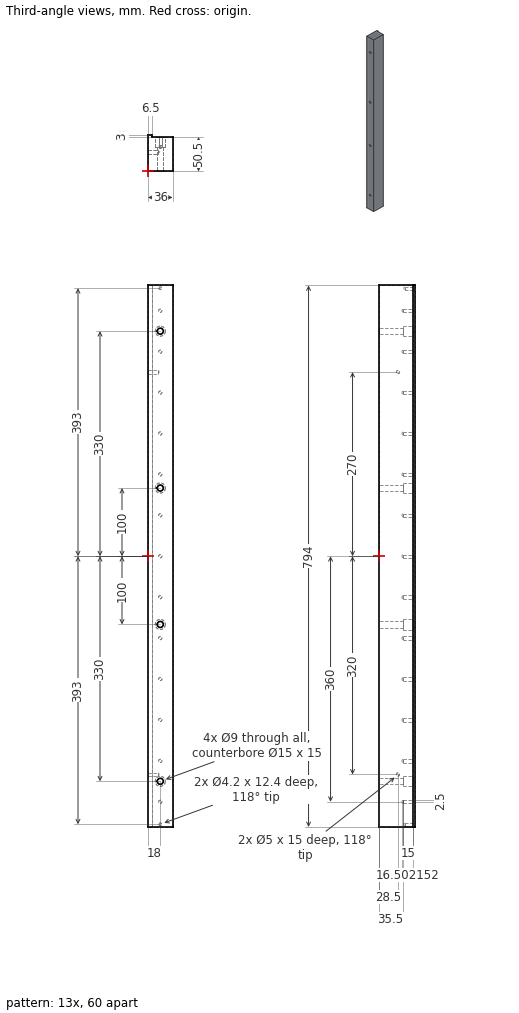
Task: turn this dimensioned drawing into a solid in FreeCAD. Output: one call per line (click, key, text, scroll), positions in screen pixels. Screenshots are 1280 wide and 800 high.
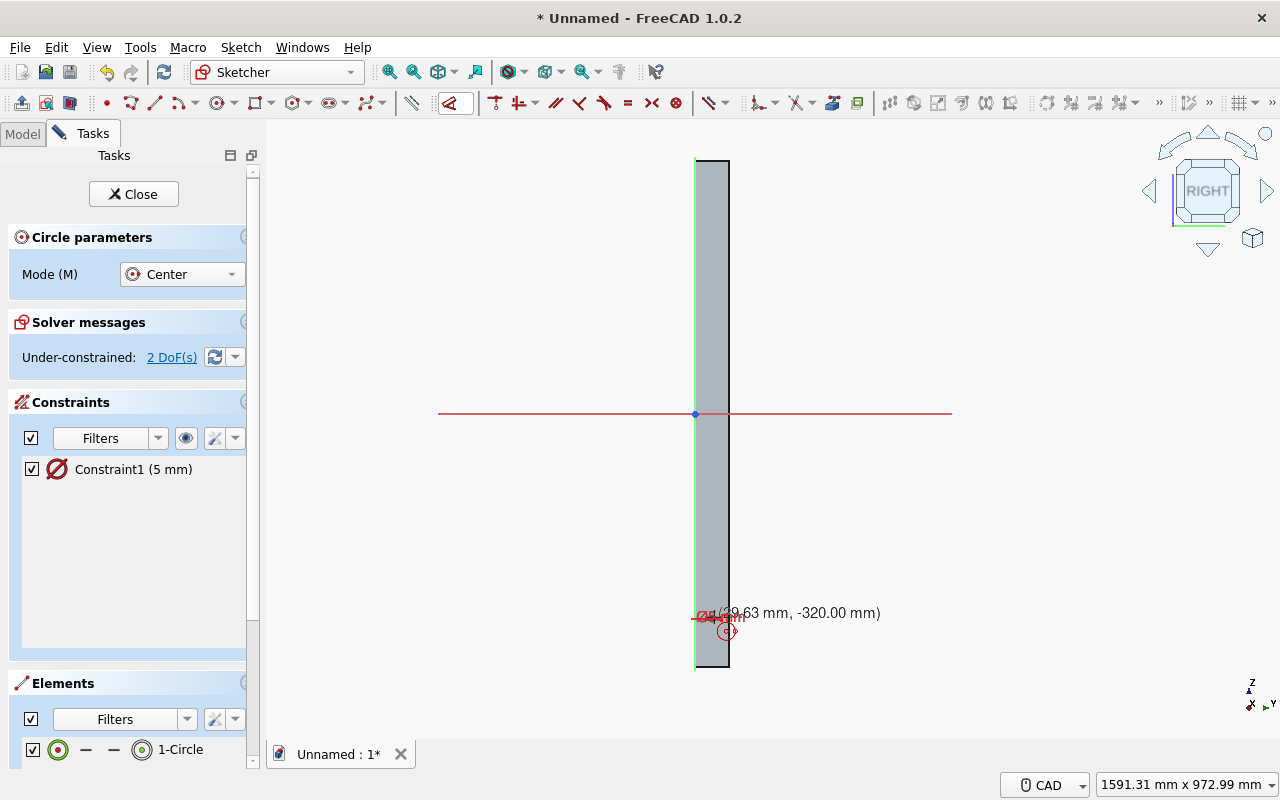
scroll(713, 242, up, 14)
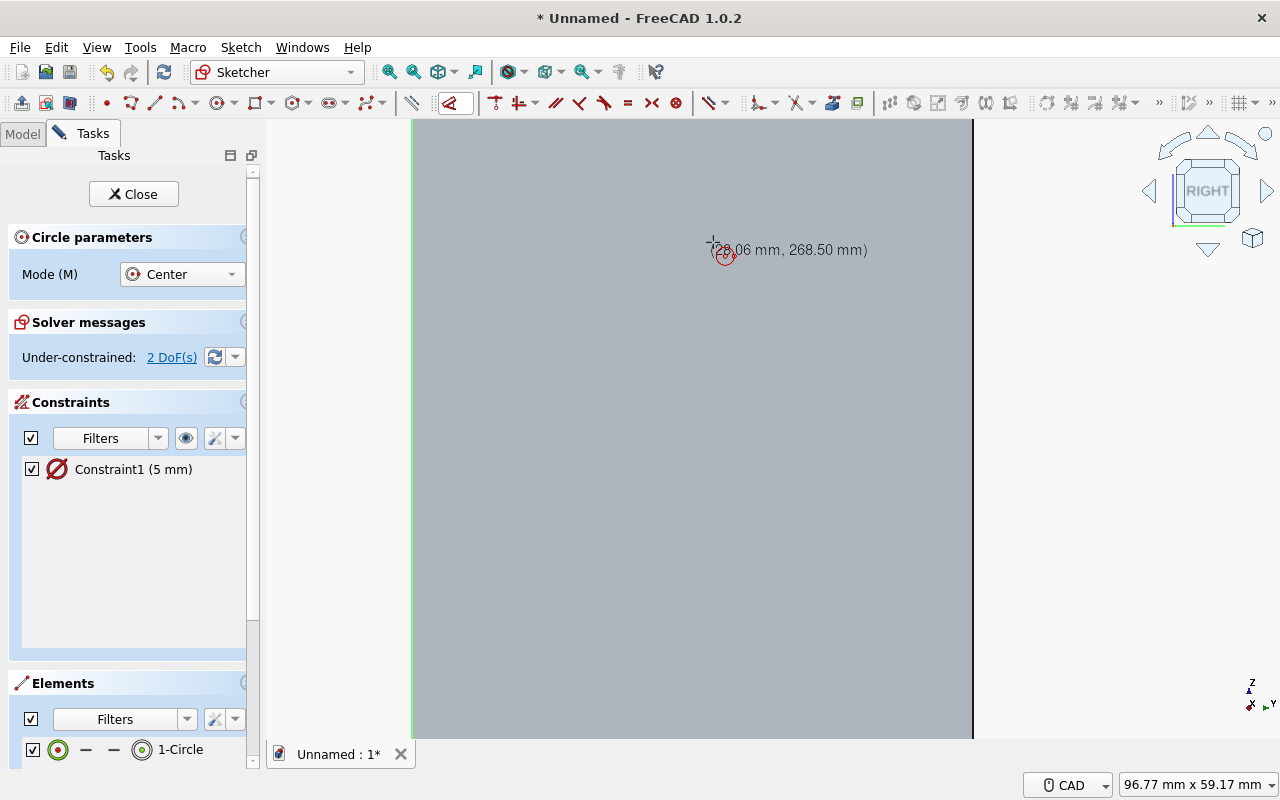
scroll(713, 241, down, 14)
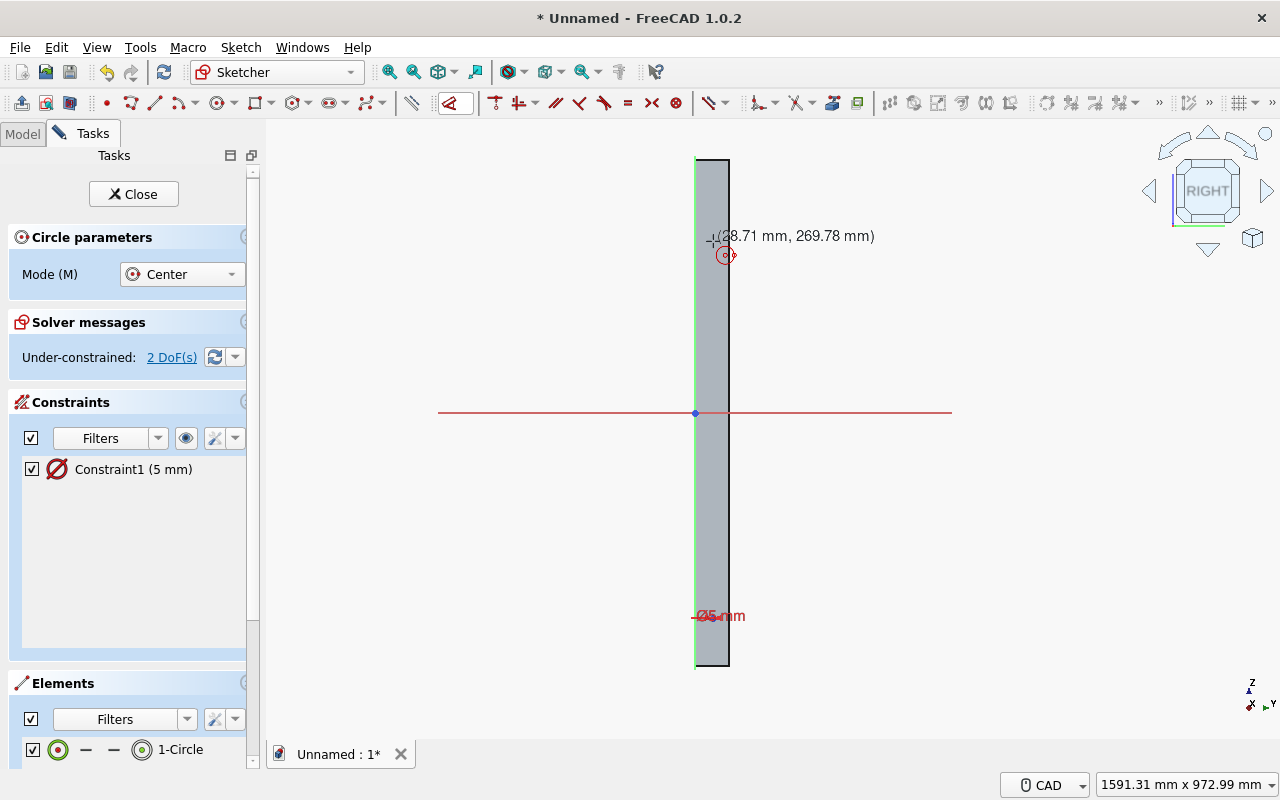
click(713, 241)
move(714, 240)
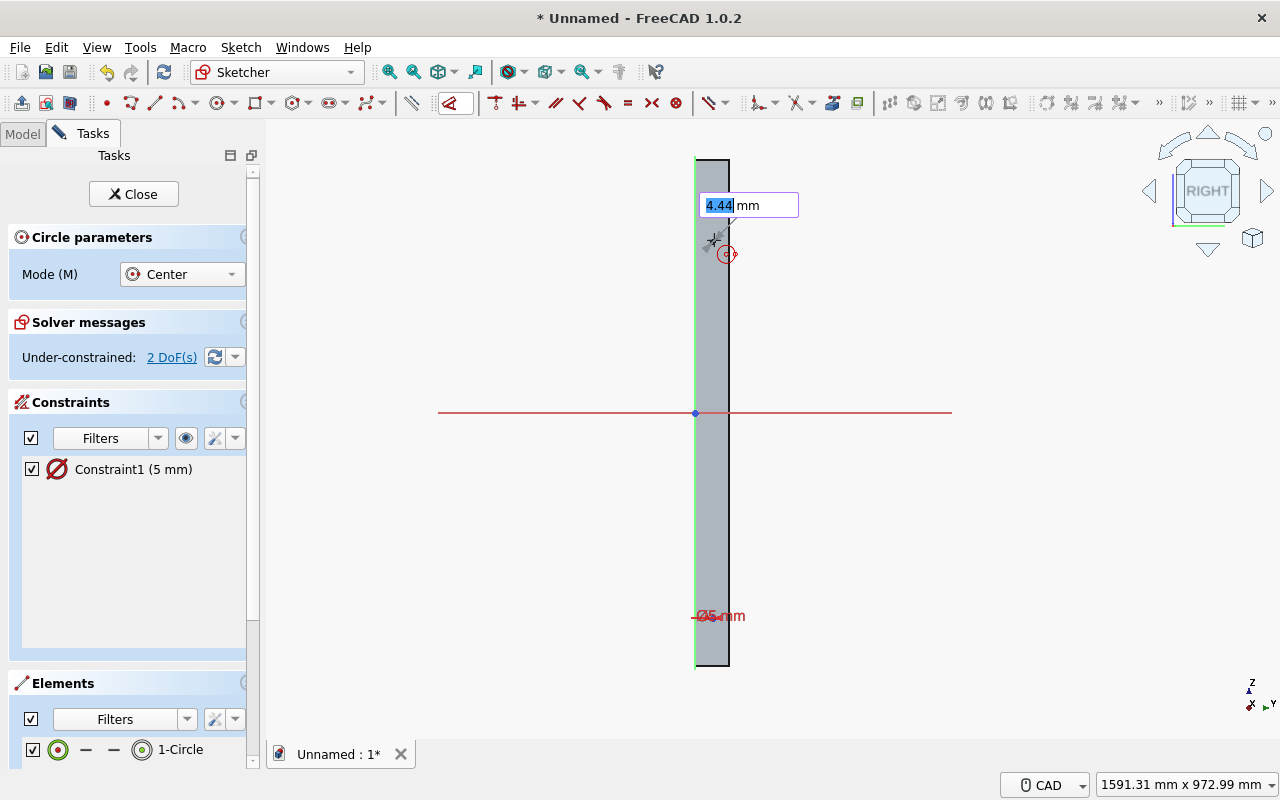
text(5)
key(Return)
key(Escape)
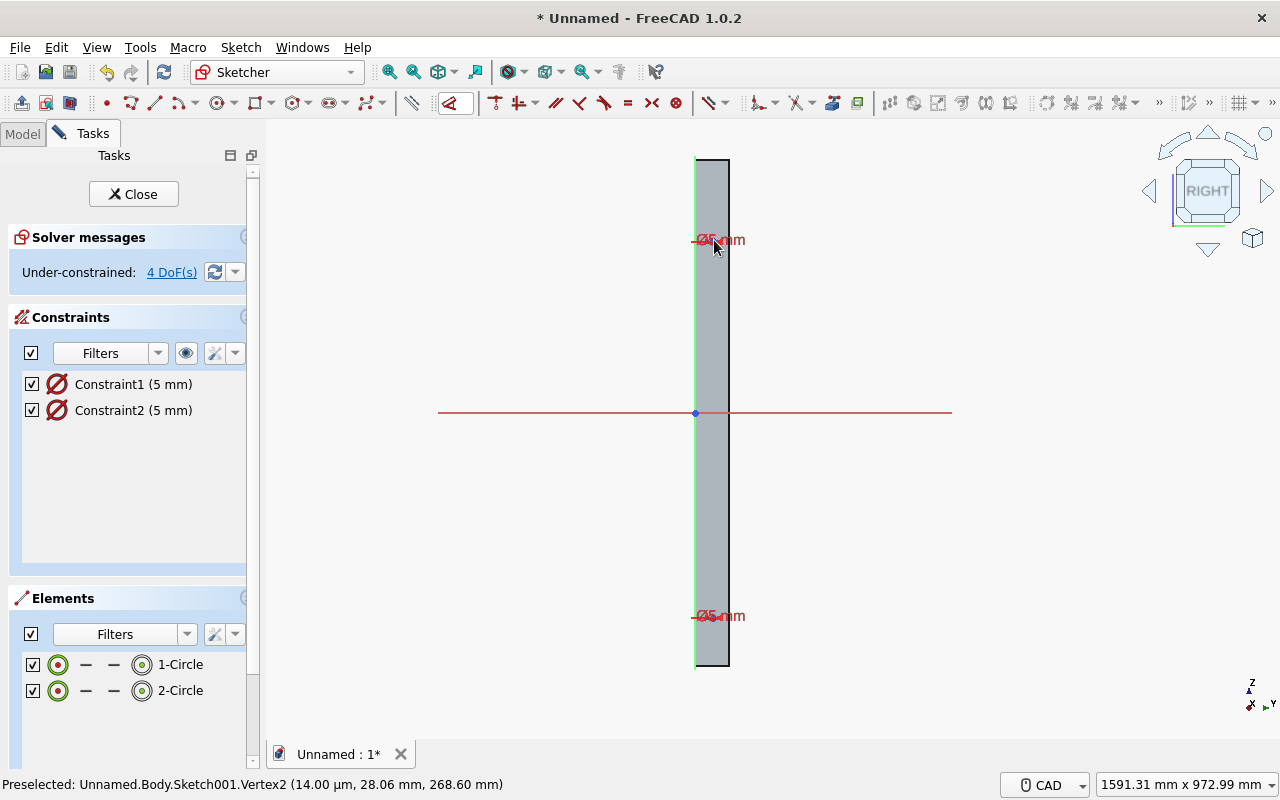
click(713, 618)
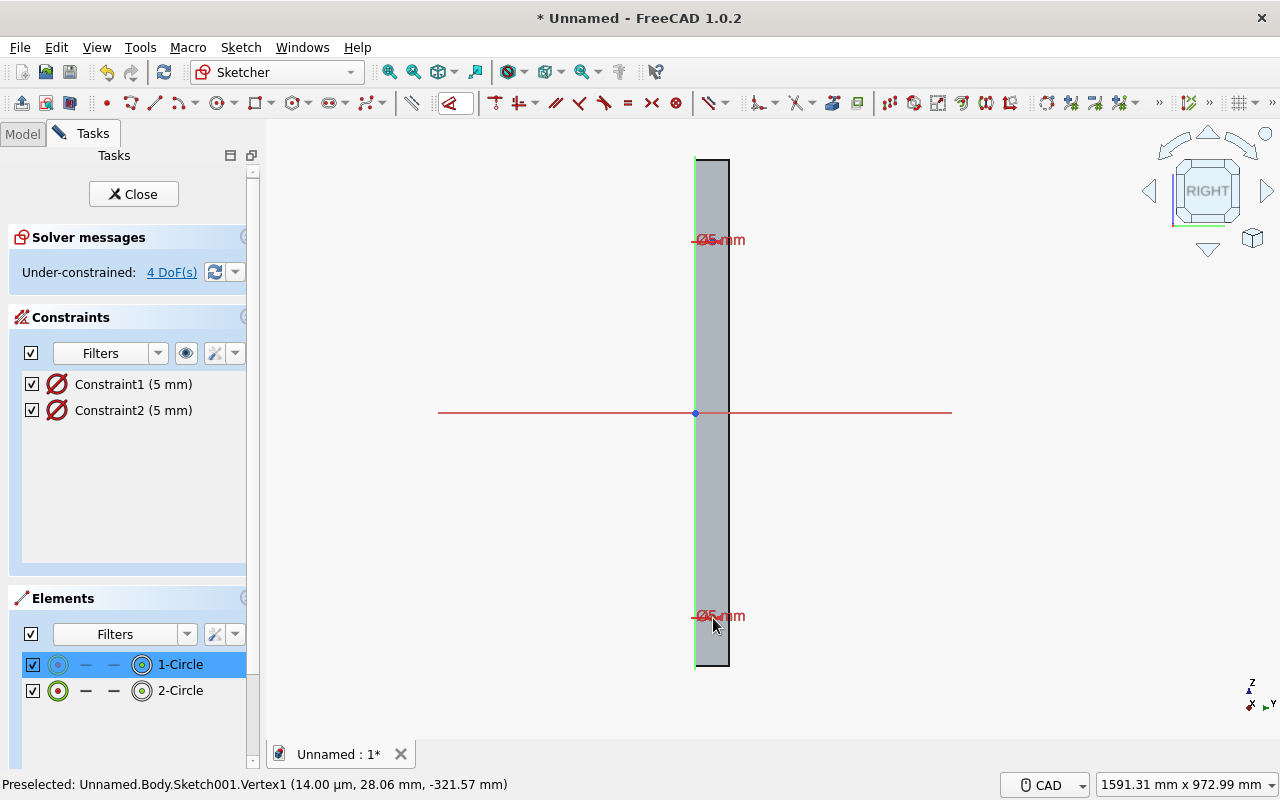
click(713, 242)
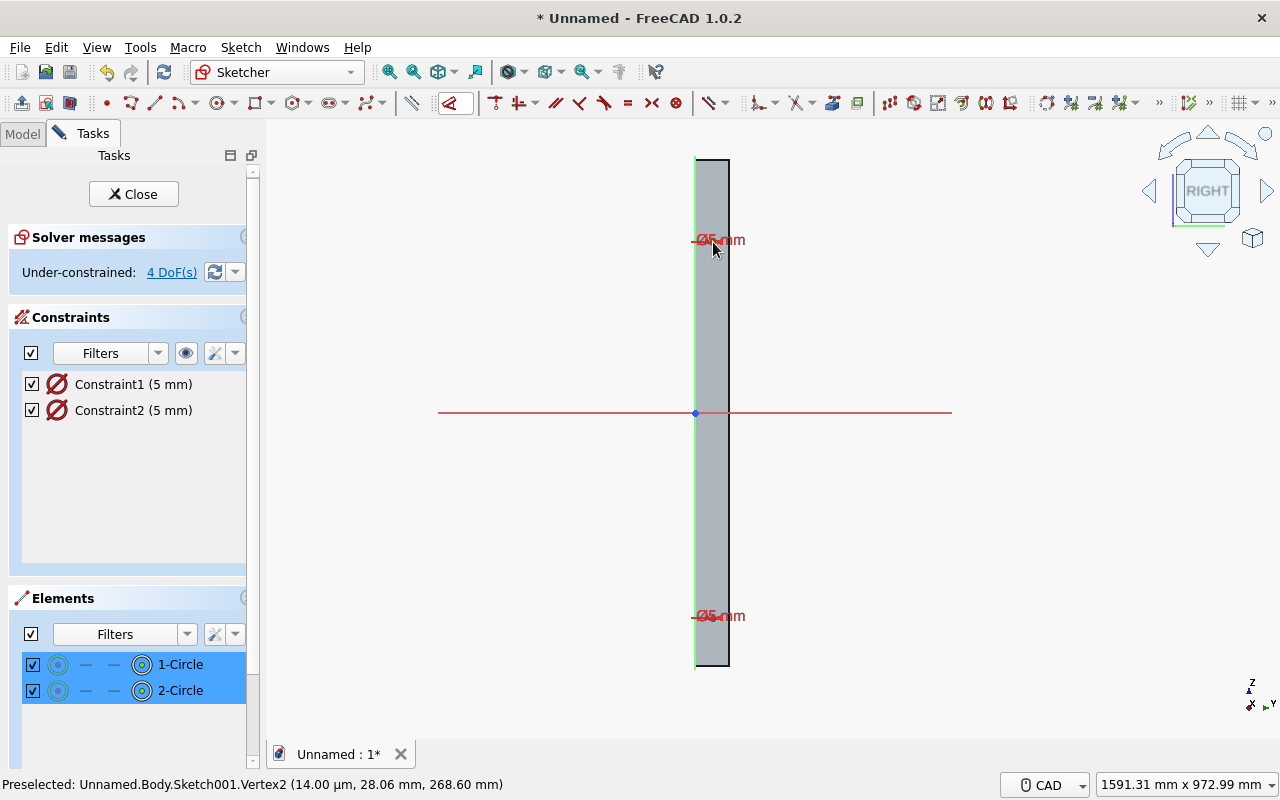
key(v)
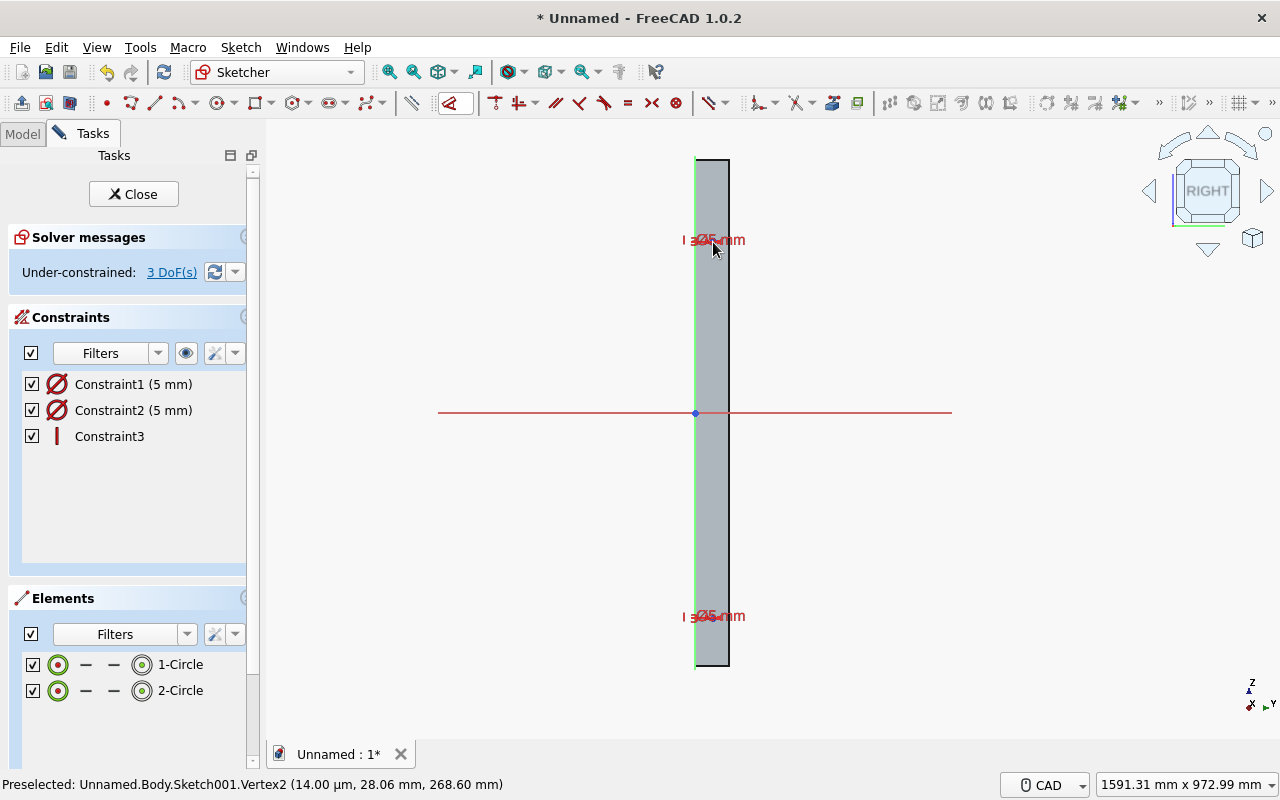
click(713, 618)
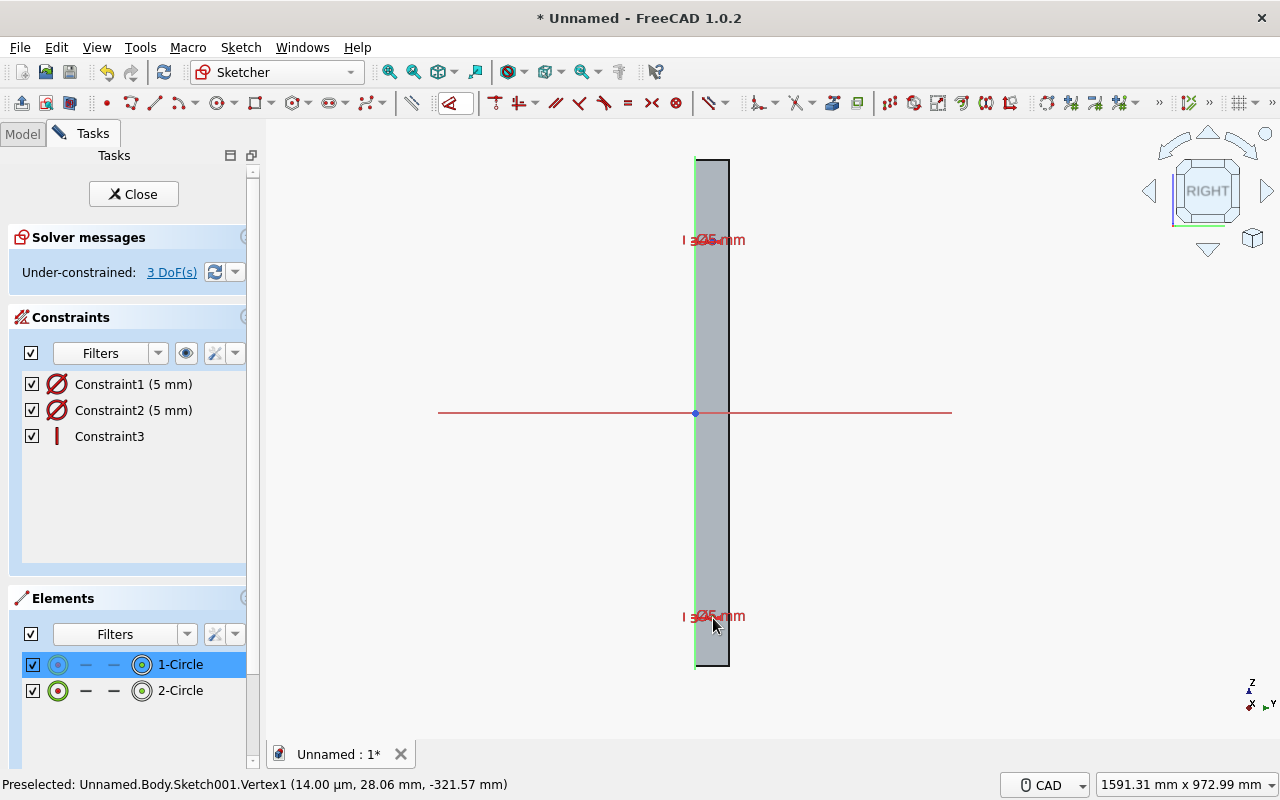
key(i)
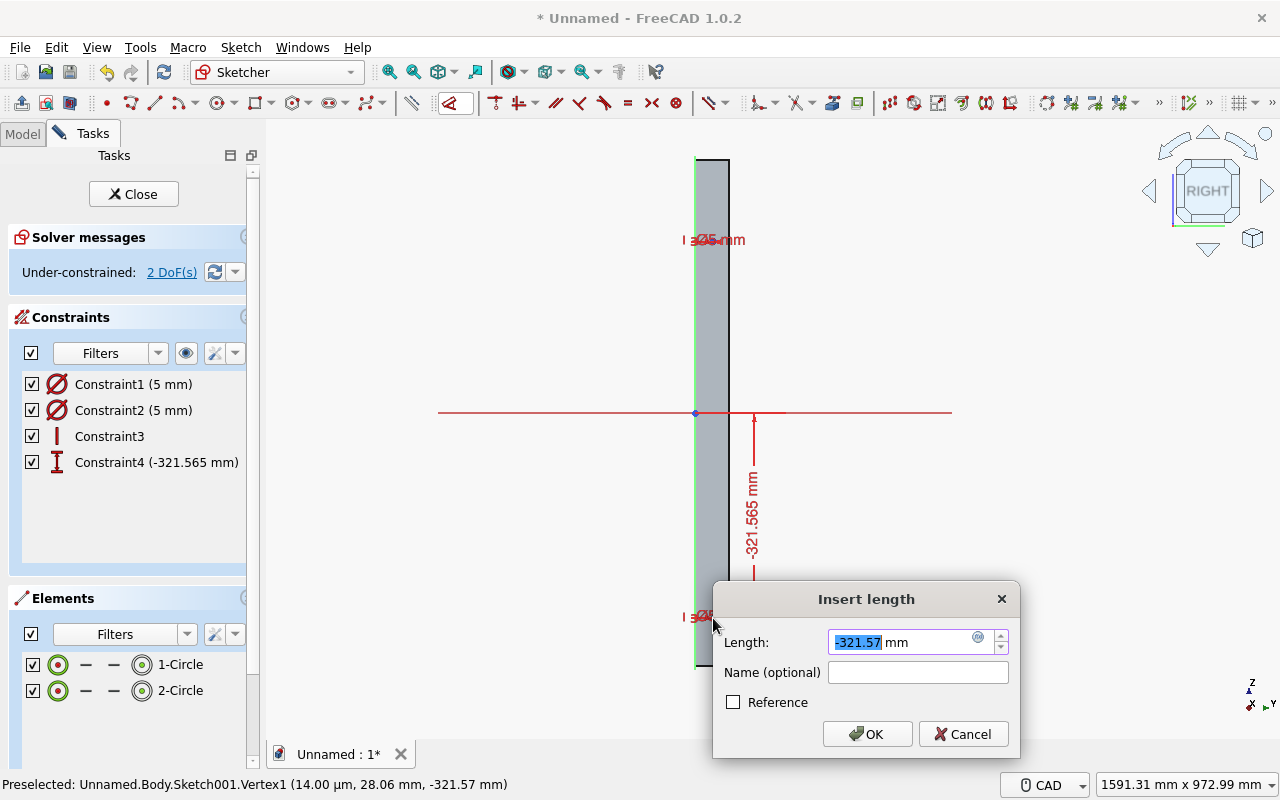
text(-320)
key(Return)